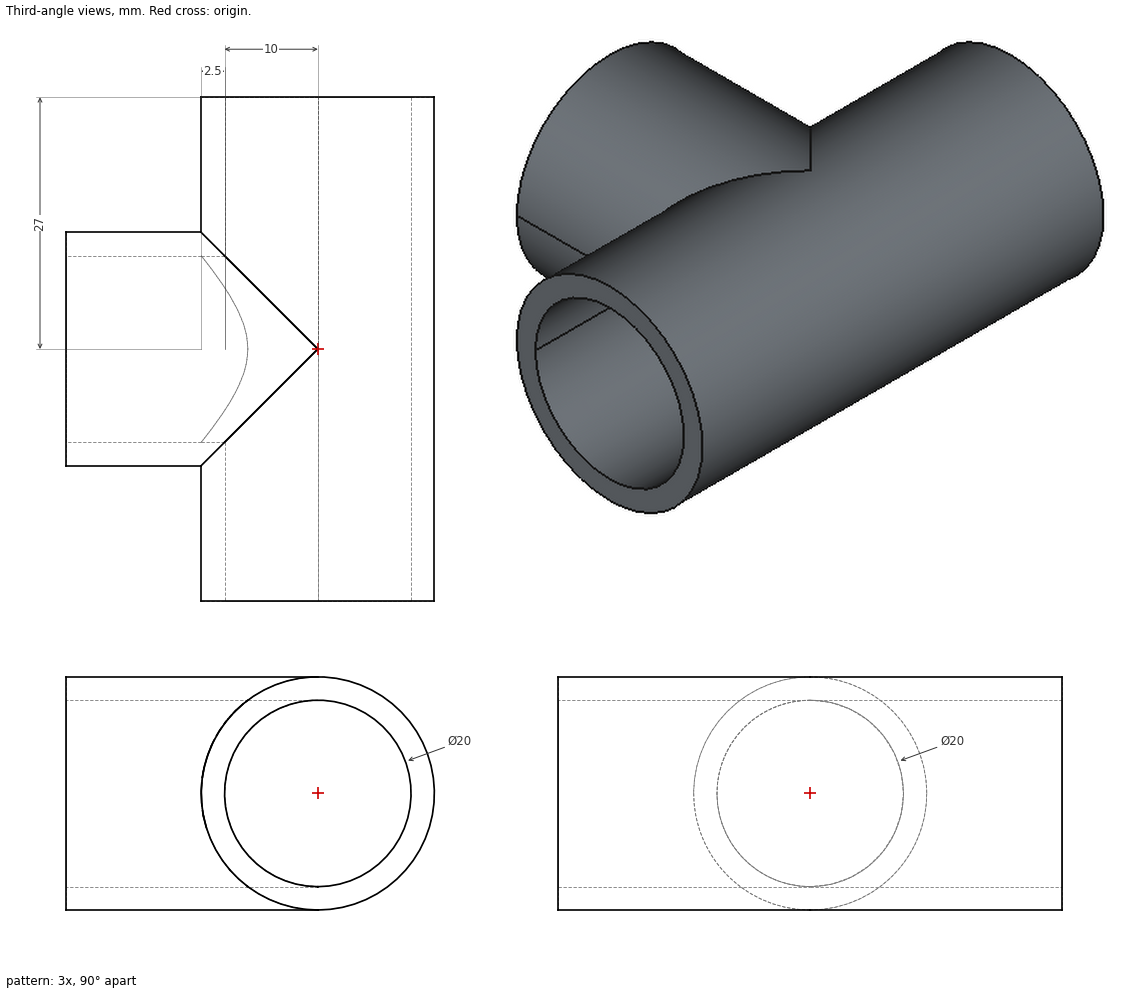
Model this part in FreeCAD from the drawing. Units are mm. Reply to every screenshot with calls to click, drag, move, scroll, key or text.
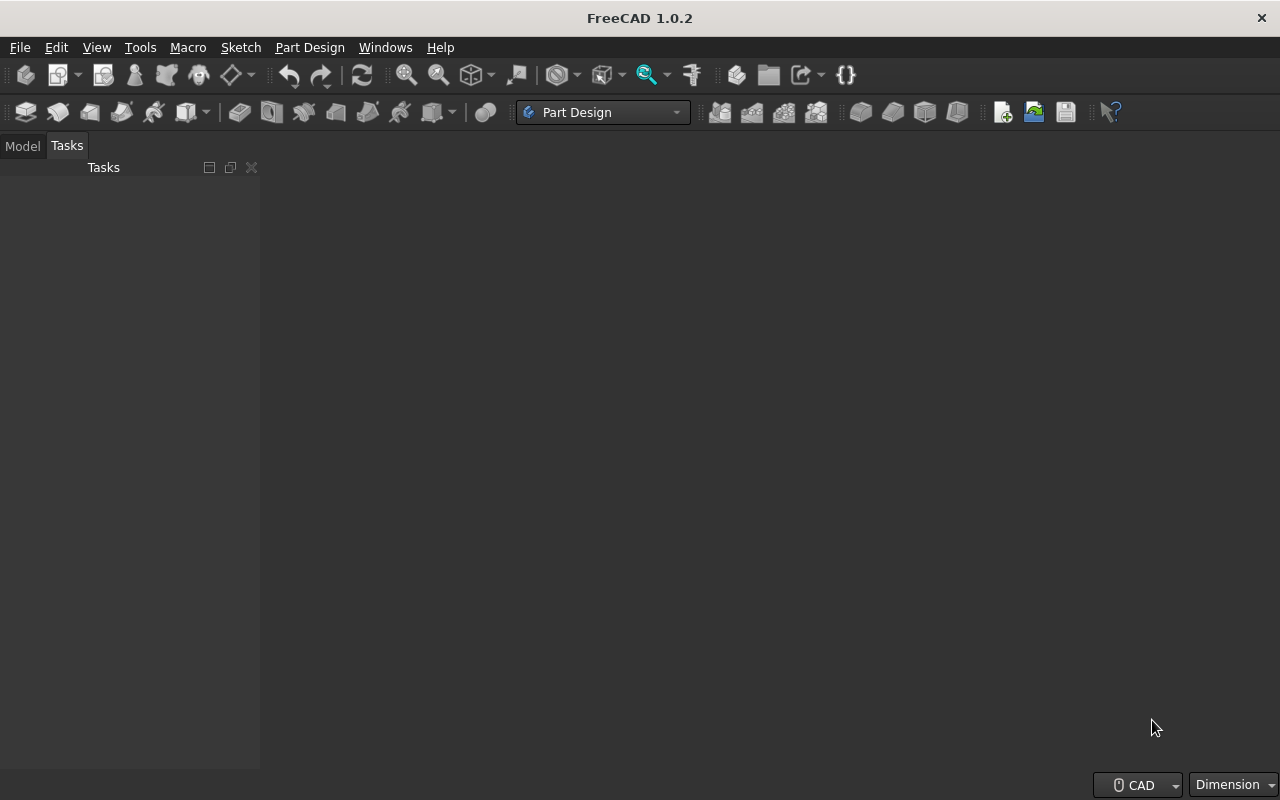
key(ctrl+n)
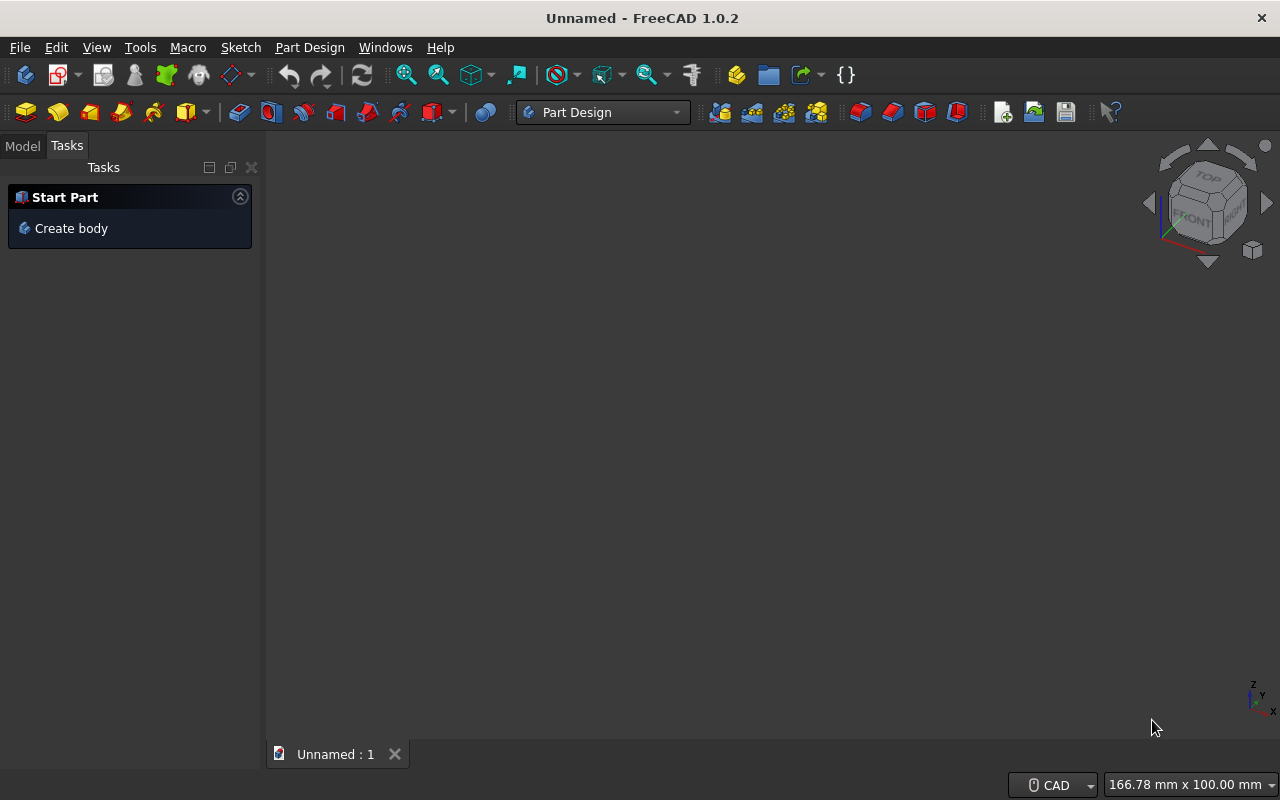
click(58, 76)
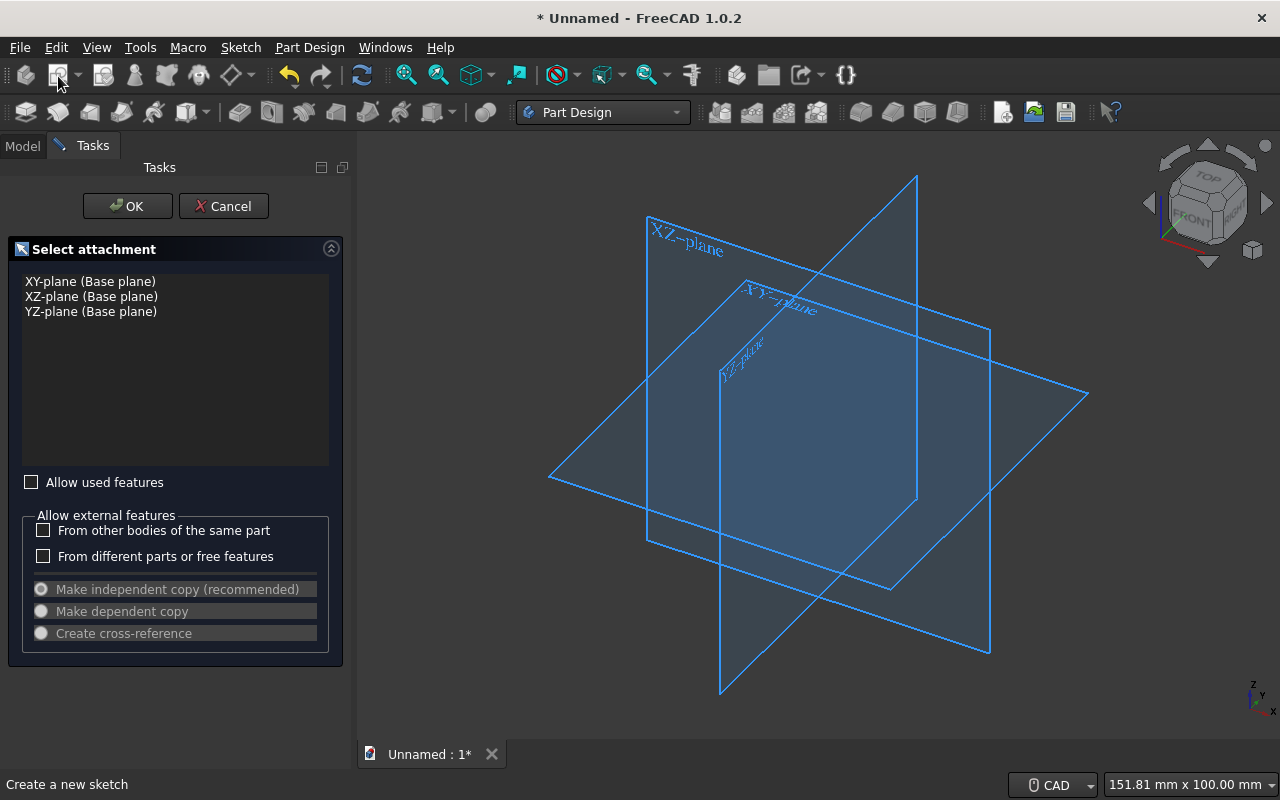
click(82, 282)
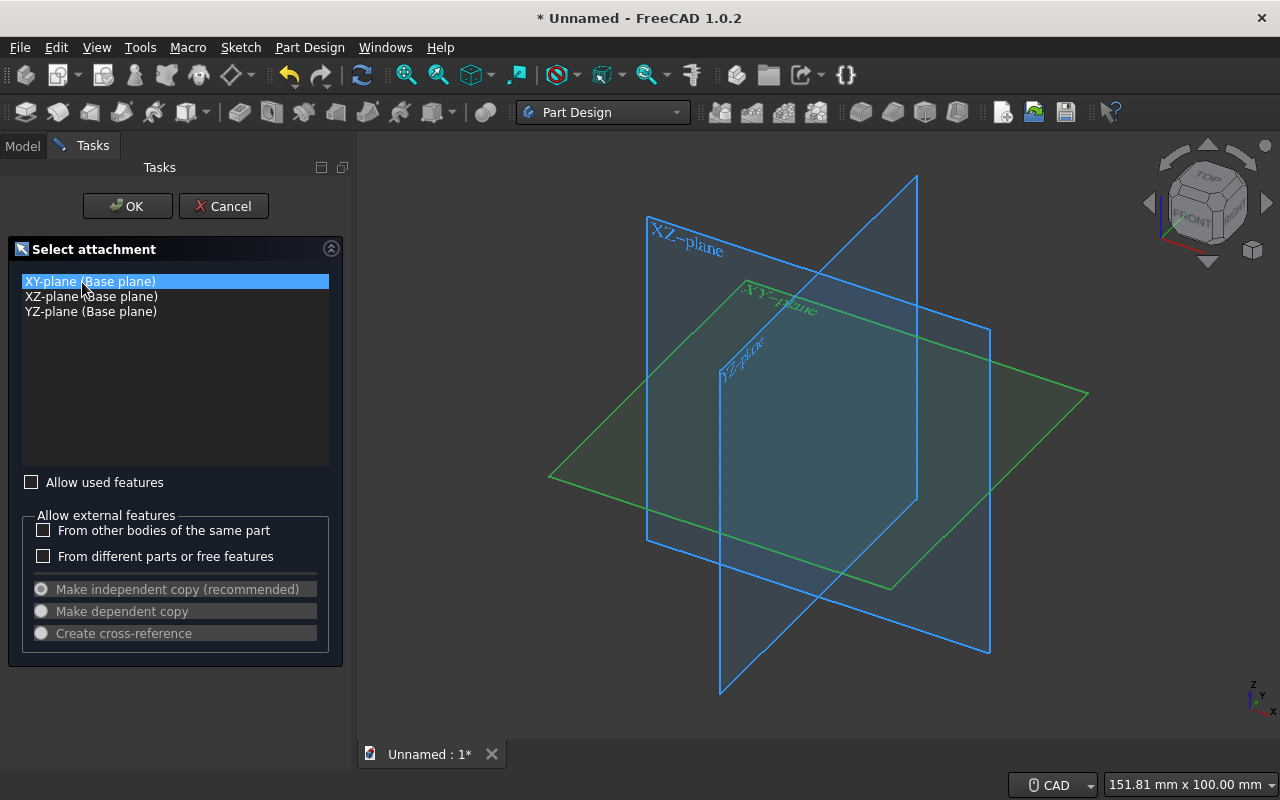
click(128, 206)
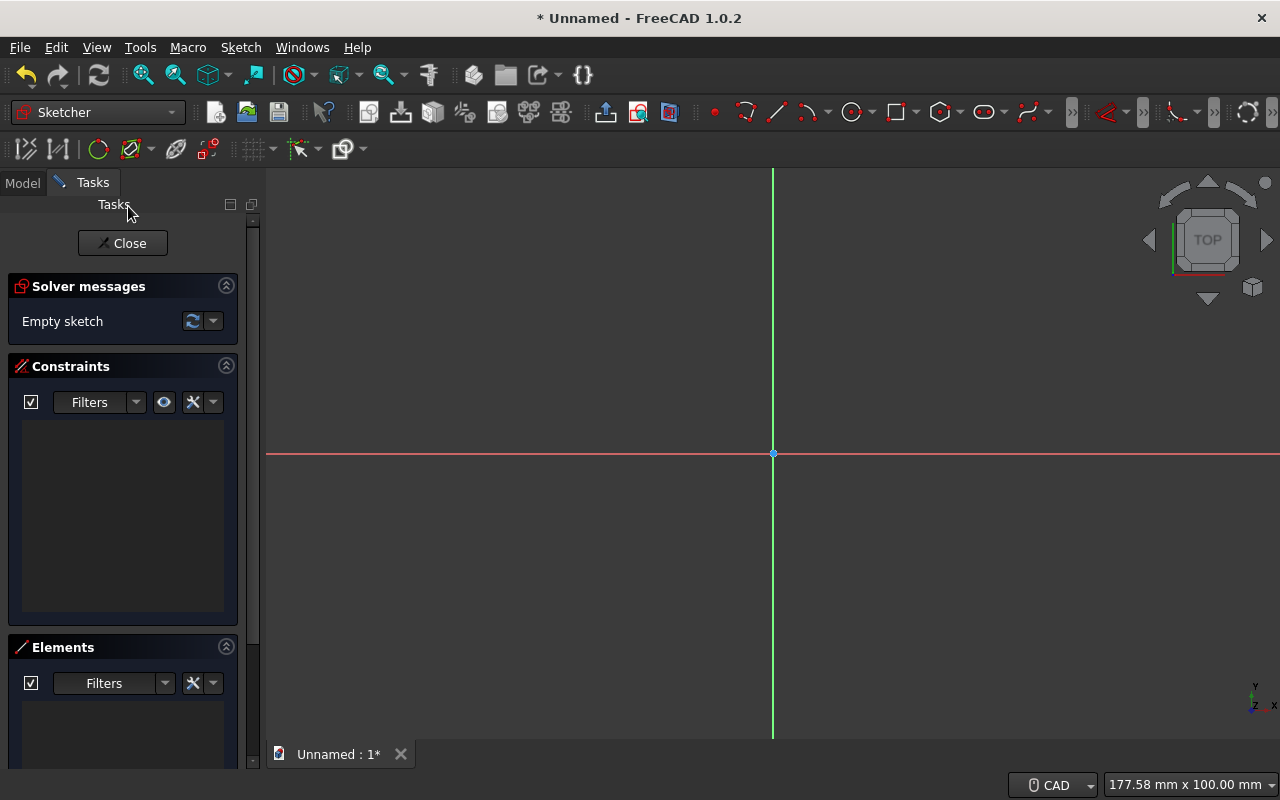
scroll(764, 314, up, 4)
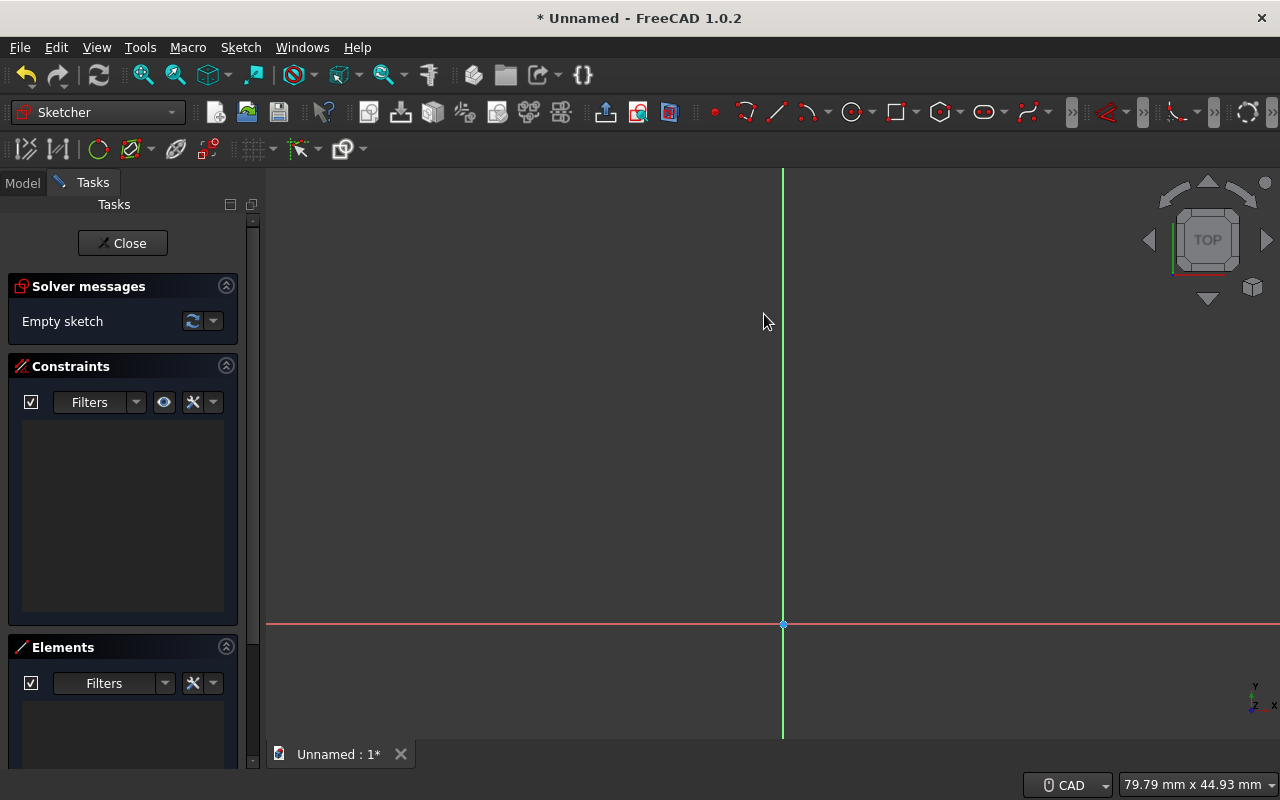
key(g)
key(r)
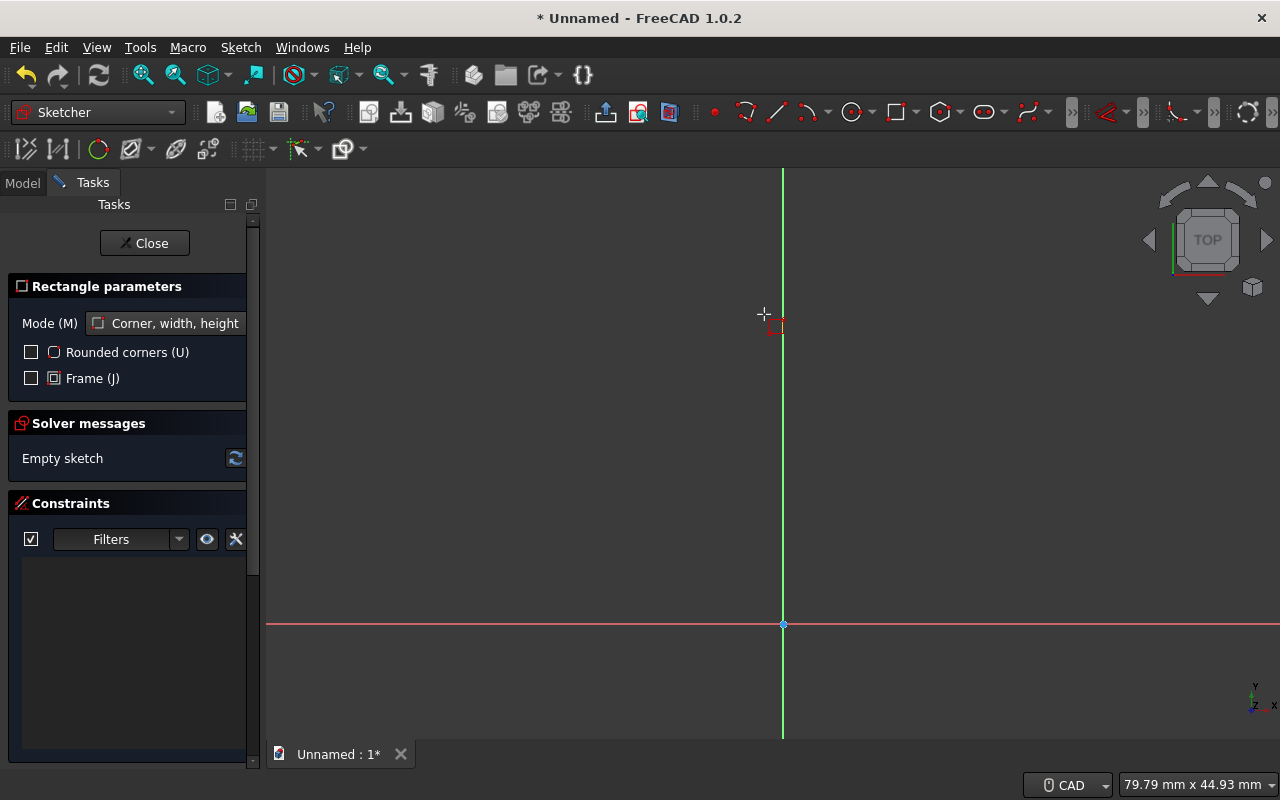
click(625, 281)
click(656, 624)
key(Escape)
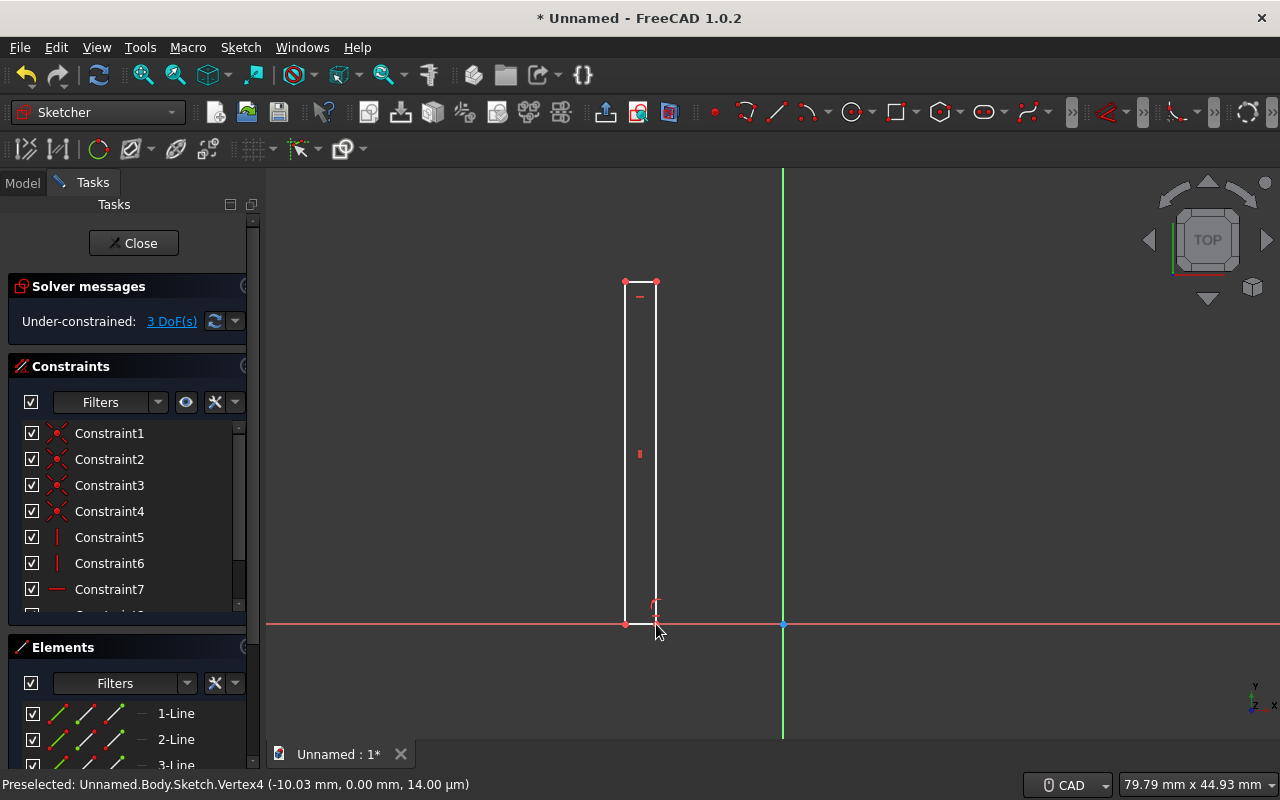
key(d)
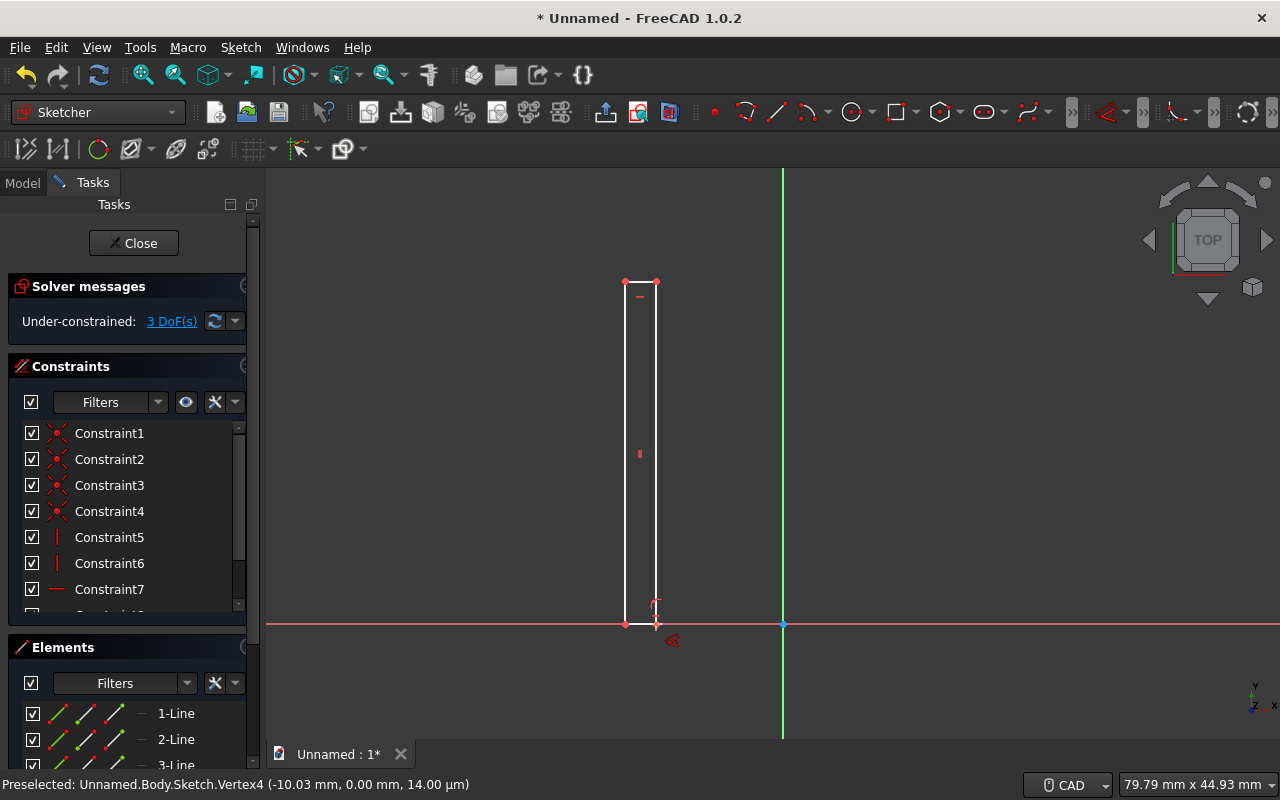
click(625, 385)
click(591, 453)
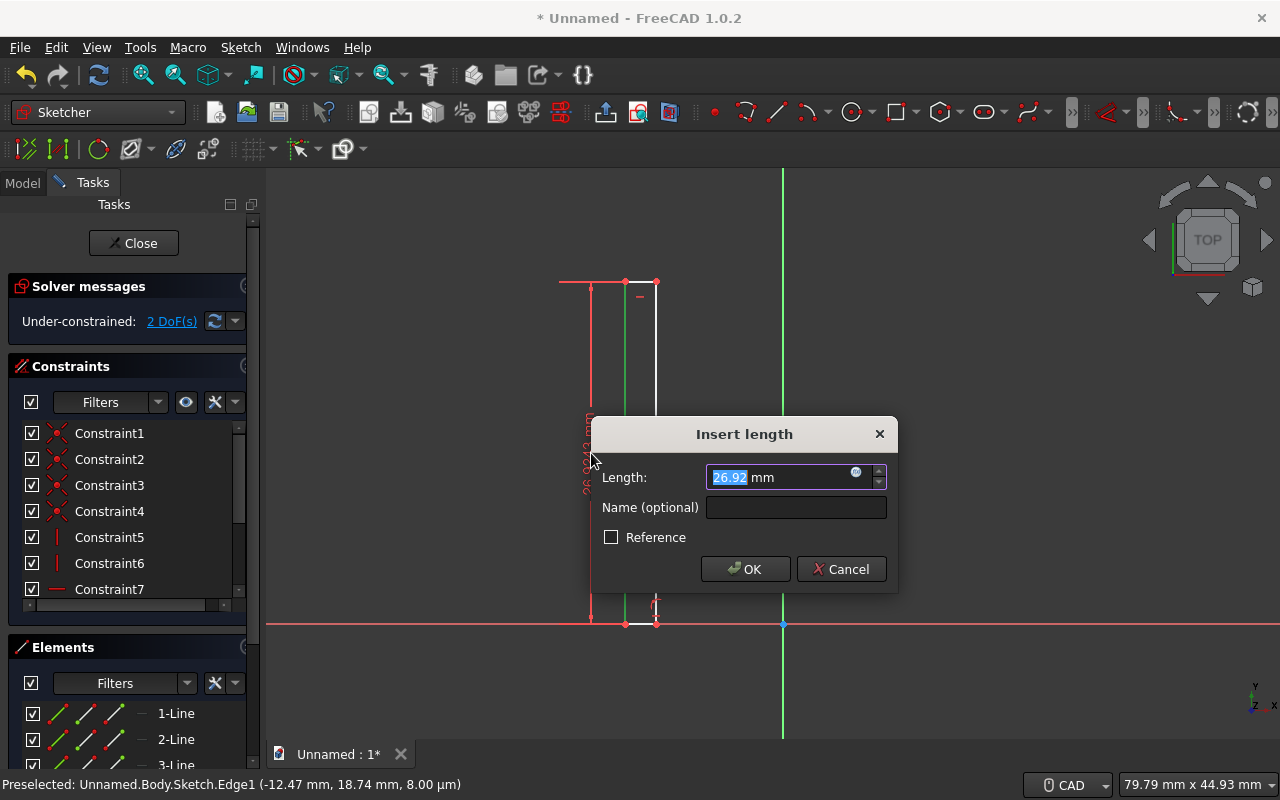
text(27)
key(Return)